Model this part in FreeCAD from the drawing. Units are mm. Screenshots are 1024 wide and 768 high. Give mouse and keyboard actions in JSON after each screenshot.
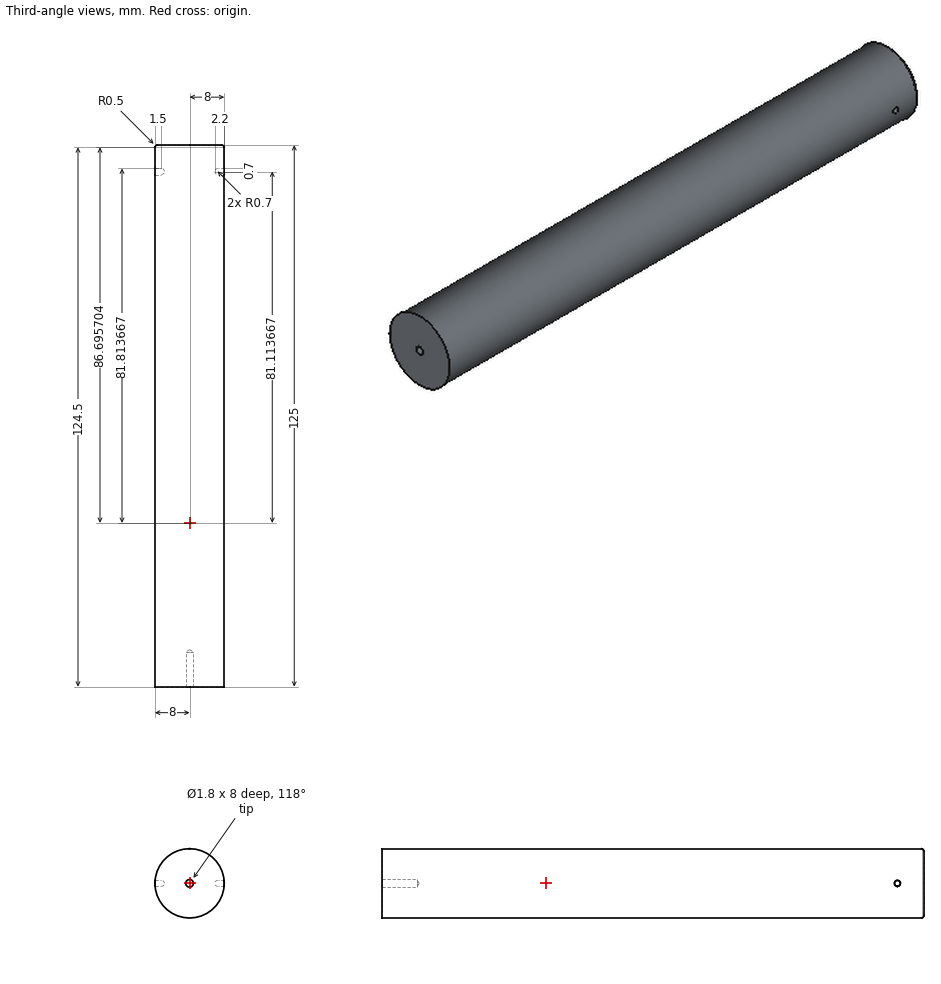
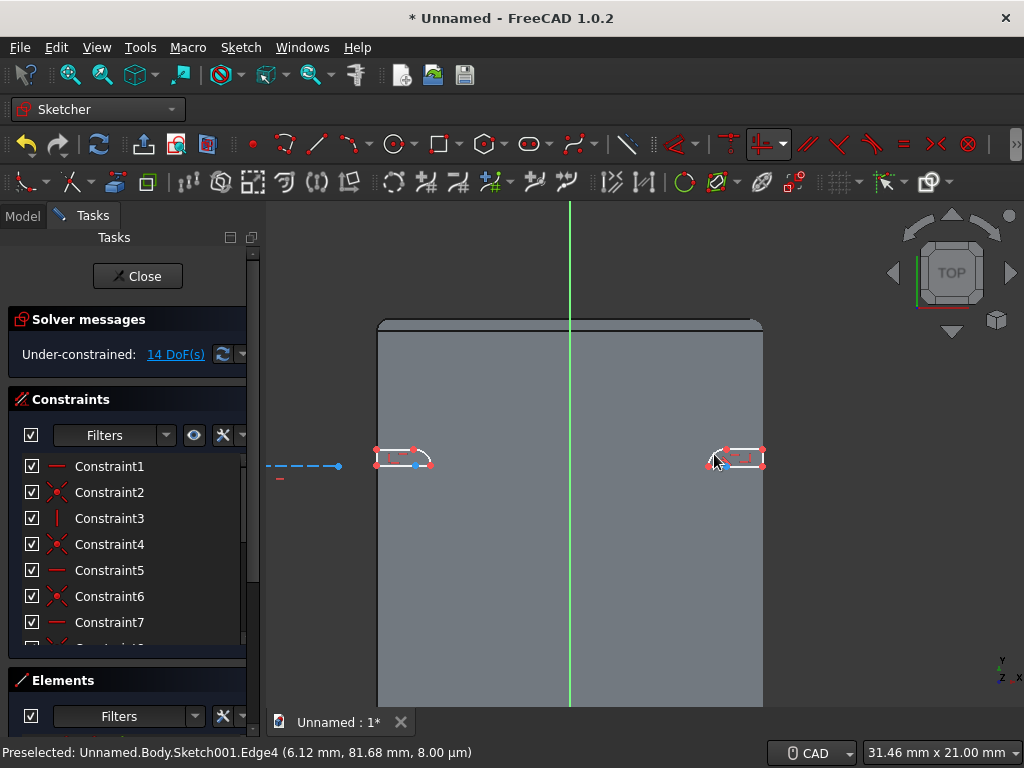
{"action": "scroll", "coordinate": [403, 450], "scroll_direction": "up", "scroll_amount": 2}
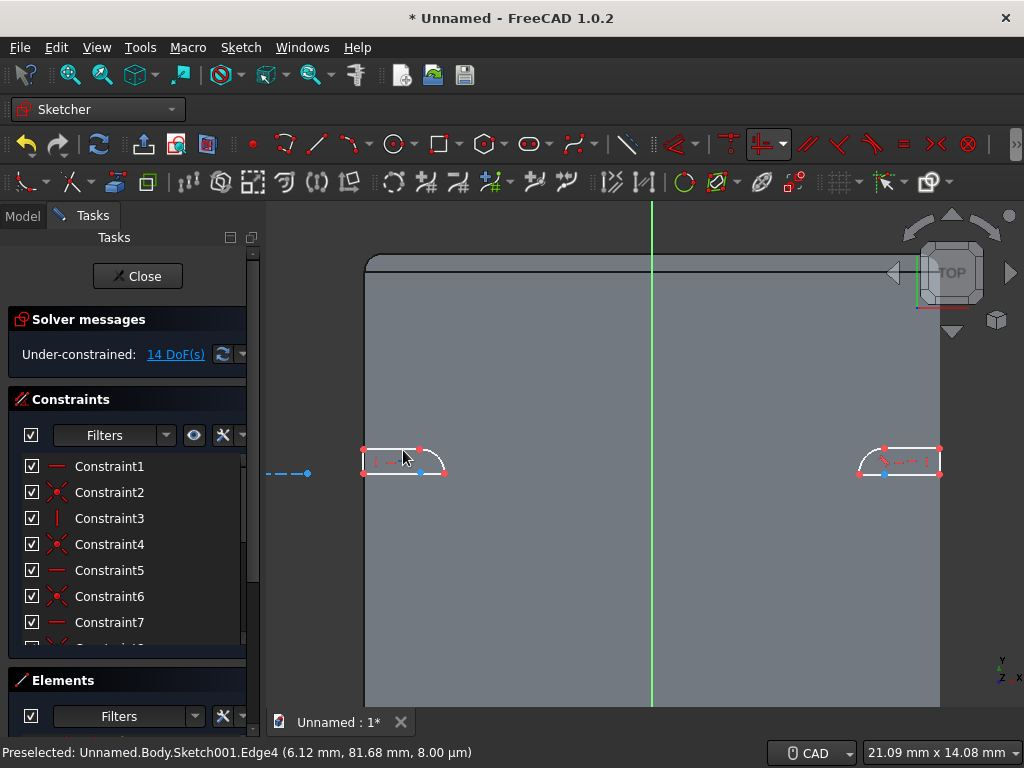
{"action": "left_click", "coordinate": [402, 449]}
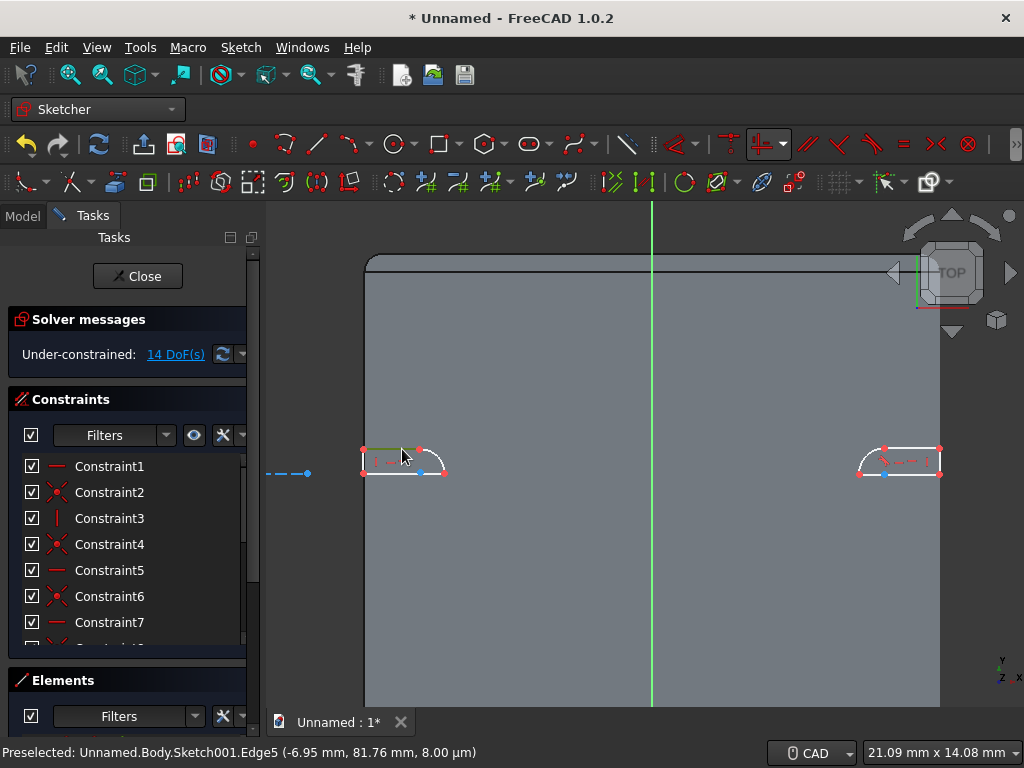
{"action": "left_click", "coordinate": [442, 462]}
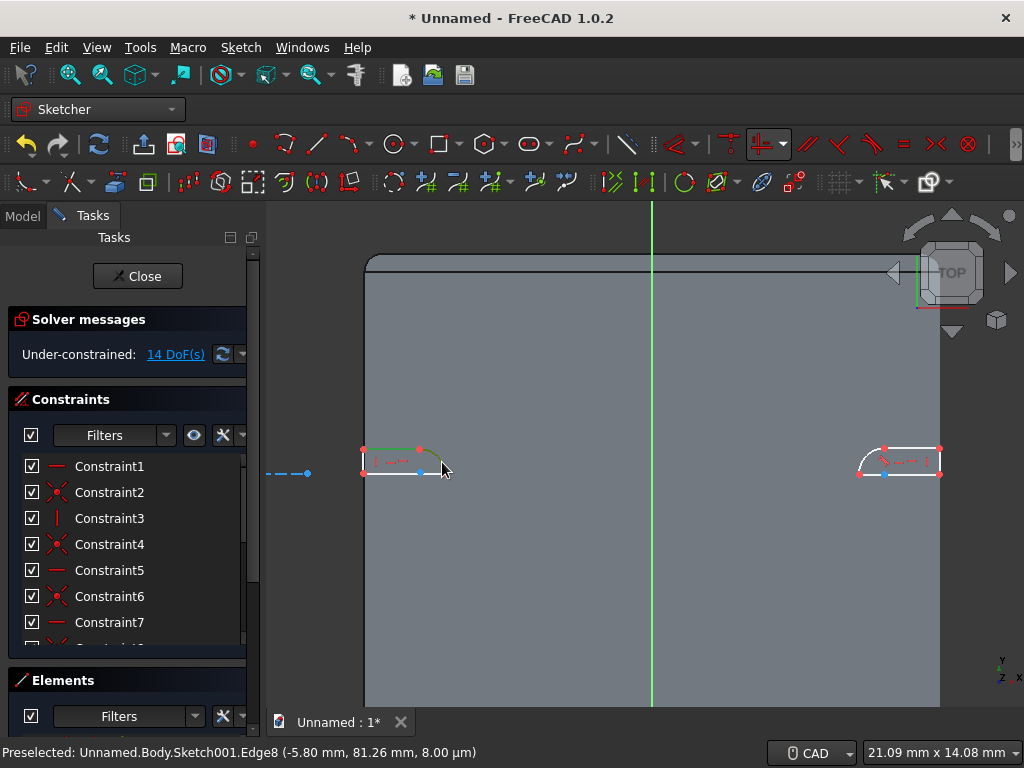
{"action": "key", "text": "t"}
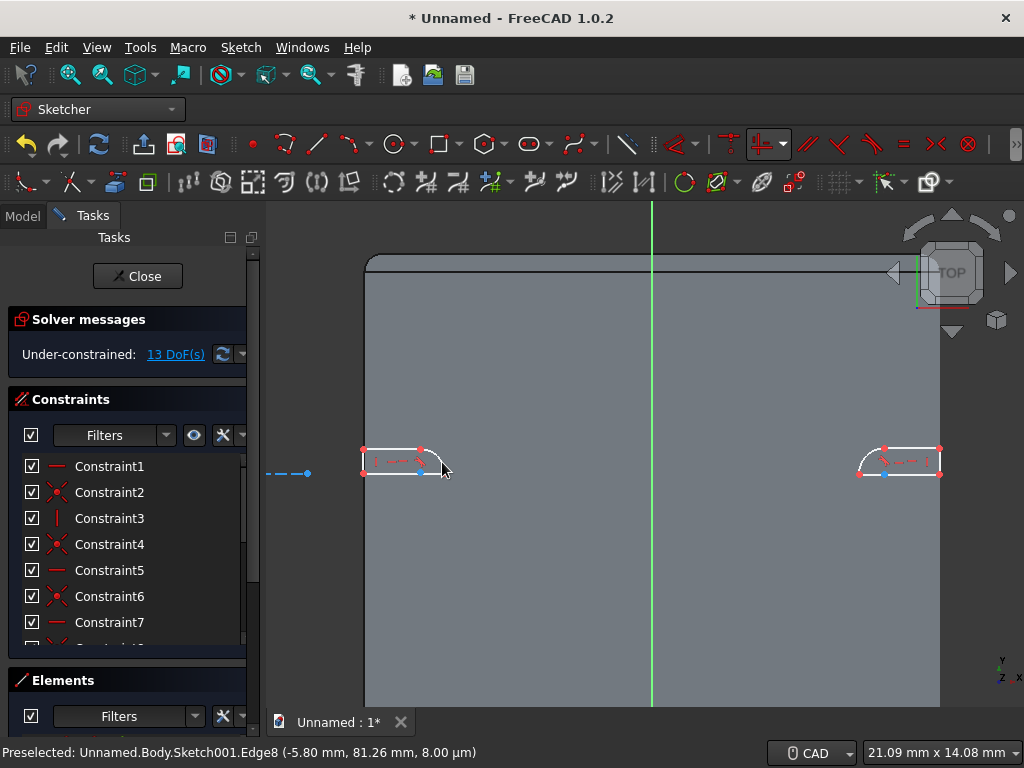
{"action": "scroll", "coordinate": [609, 449], "scroll_direction": "down", "scroll_amount": 4}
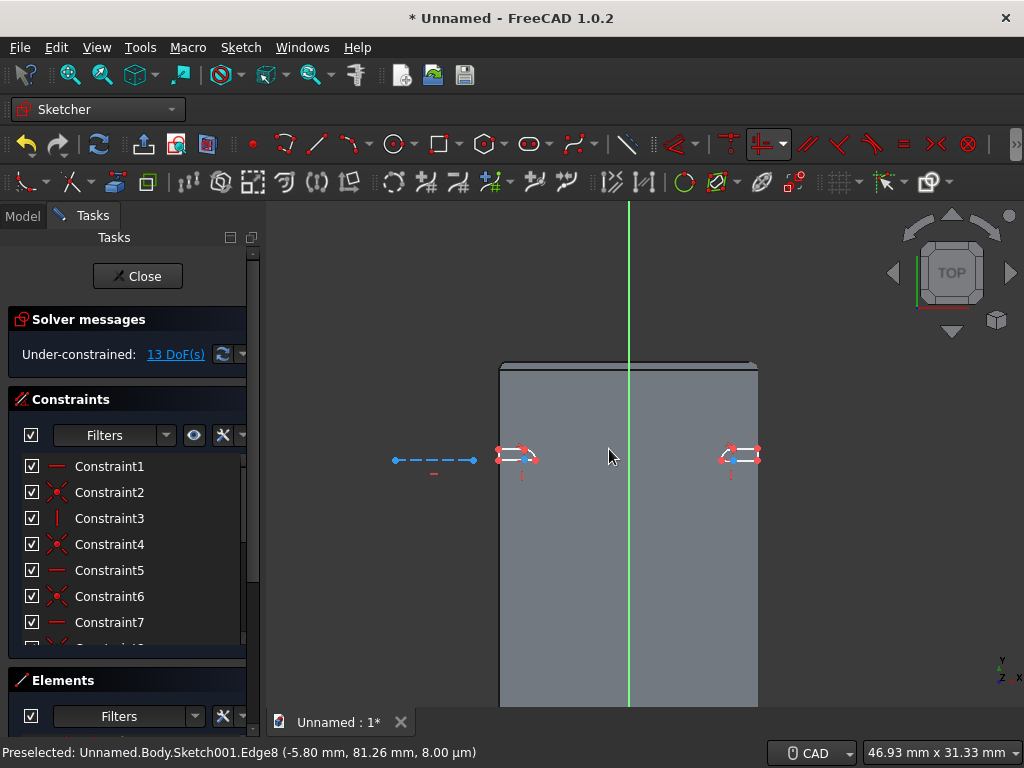
{"action": "scroll", "coordinate": [728, 450], "scroll_direction": "up", "scroll_amount": 5}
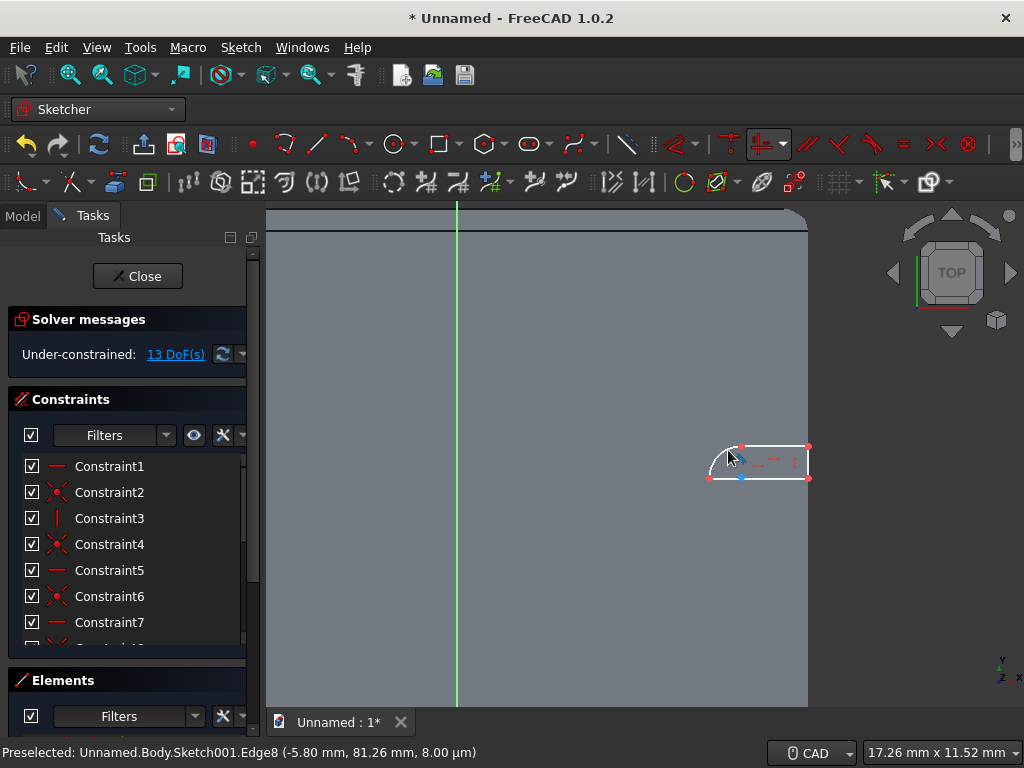
{"action": "left_click", "coordinate": [727, 450]}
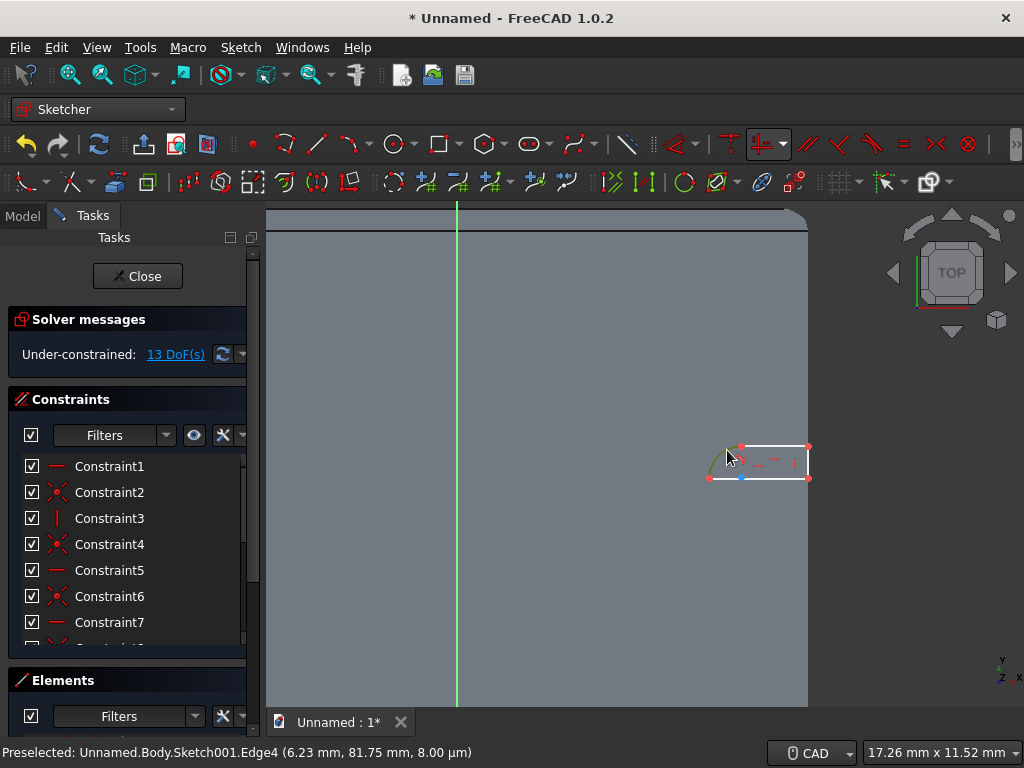
{"action": "scroll", "coordinate": [728, 450], "scroll_direction": "down", "scroll_amount": 5}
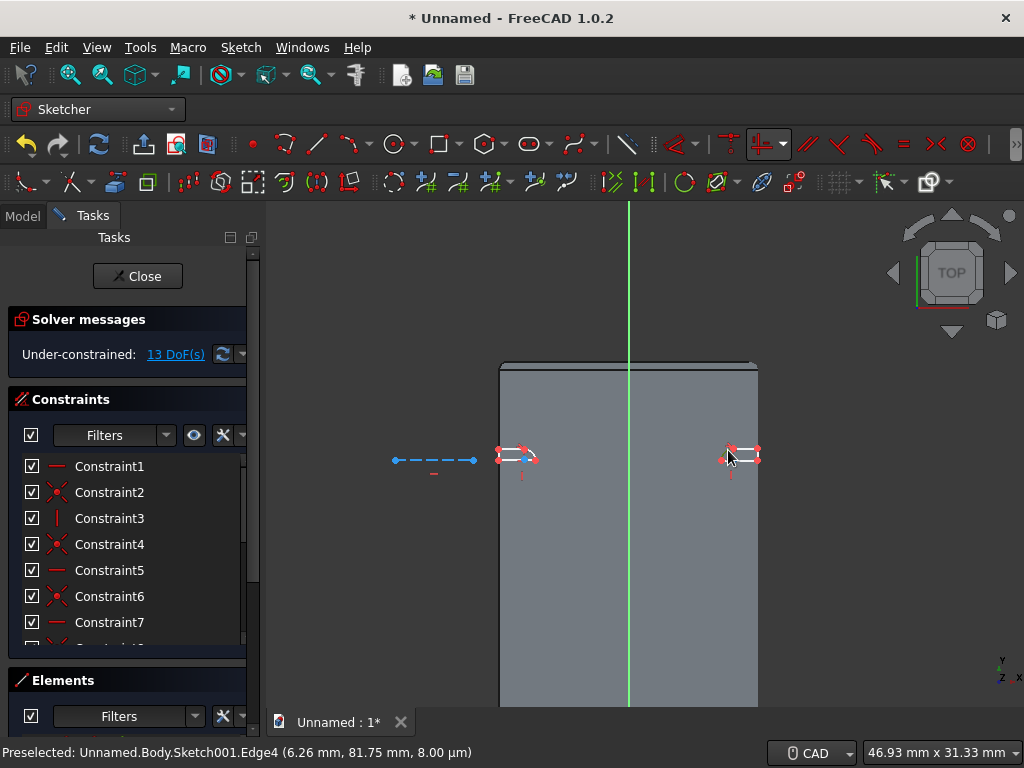
{"action": "scroll", "coordinate": [534, 455], "scroll_direction": "up", "scroll_amount": 6}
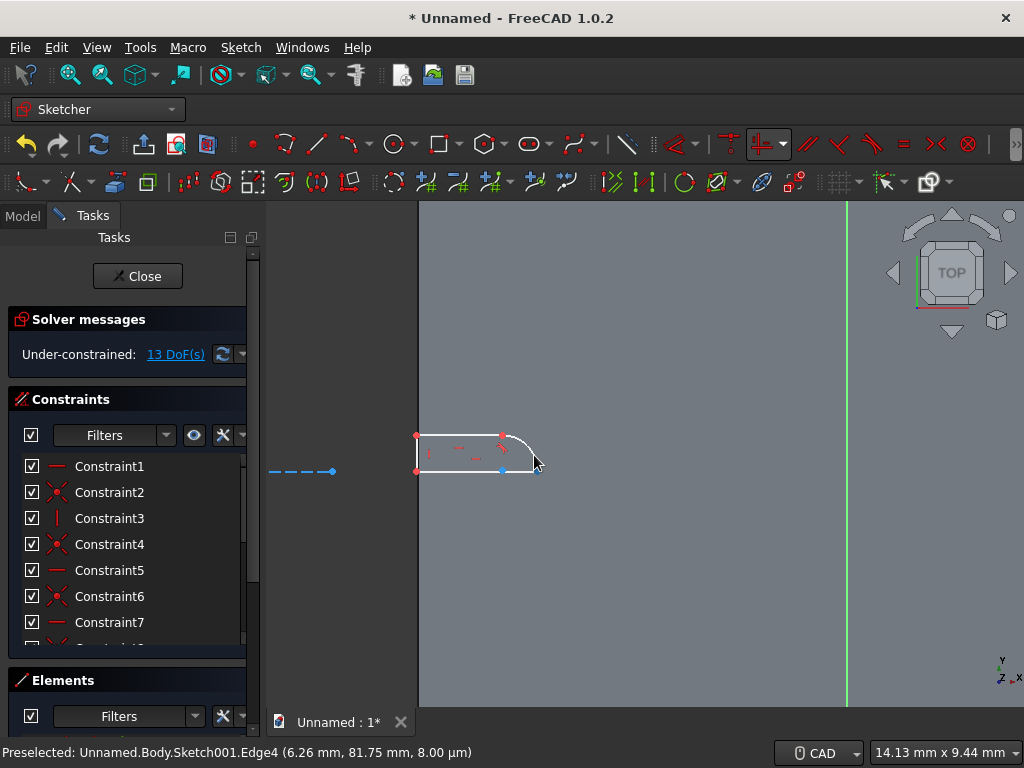
{"action": "left_click", "coordinate": [534, 455]}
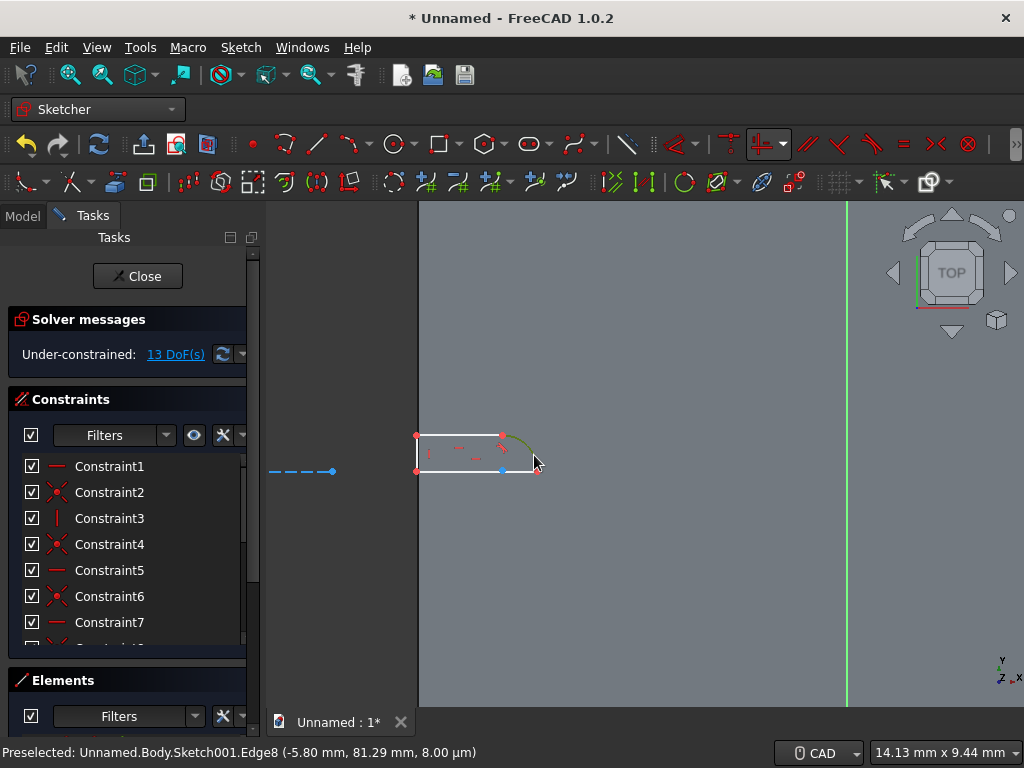
{"action": "key", "text": "e"}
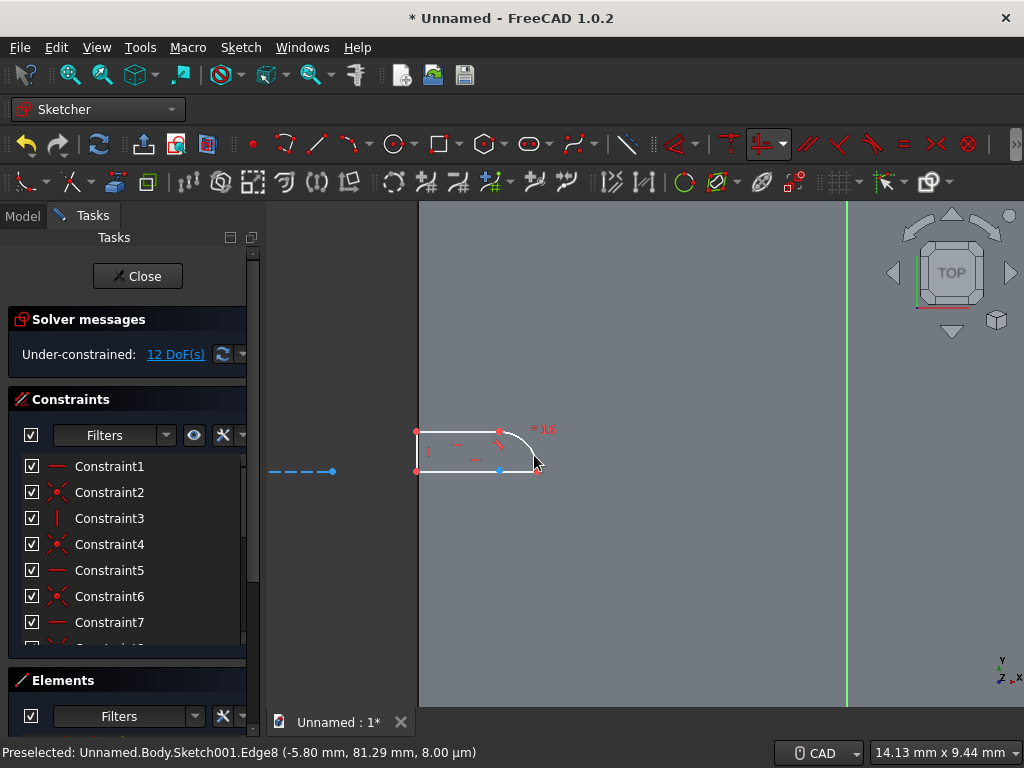
{"action": "scroll", "coordinate": [534, 455], "scroll_direction": "down", "scroll_amount": 6}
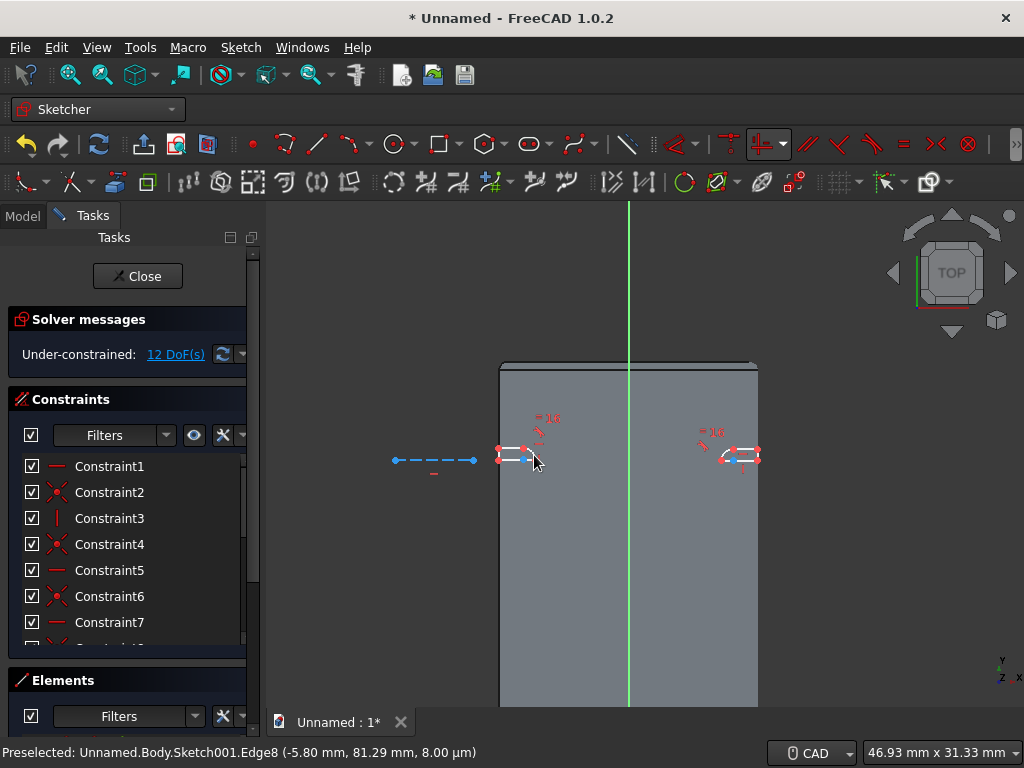
{"action": "scroll", "coordinate": [728, 450], "scroll_direction": "up", "scroll_amount": 7}